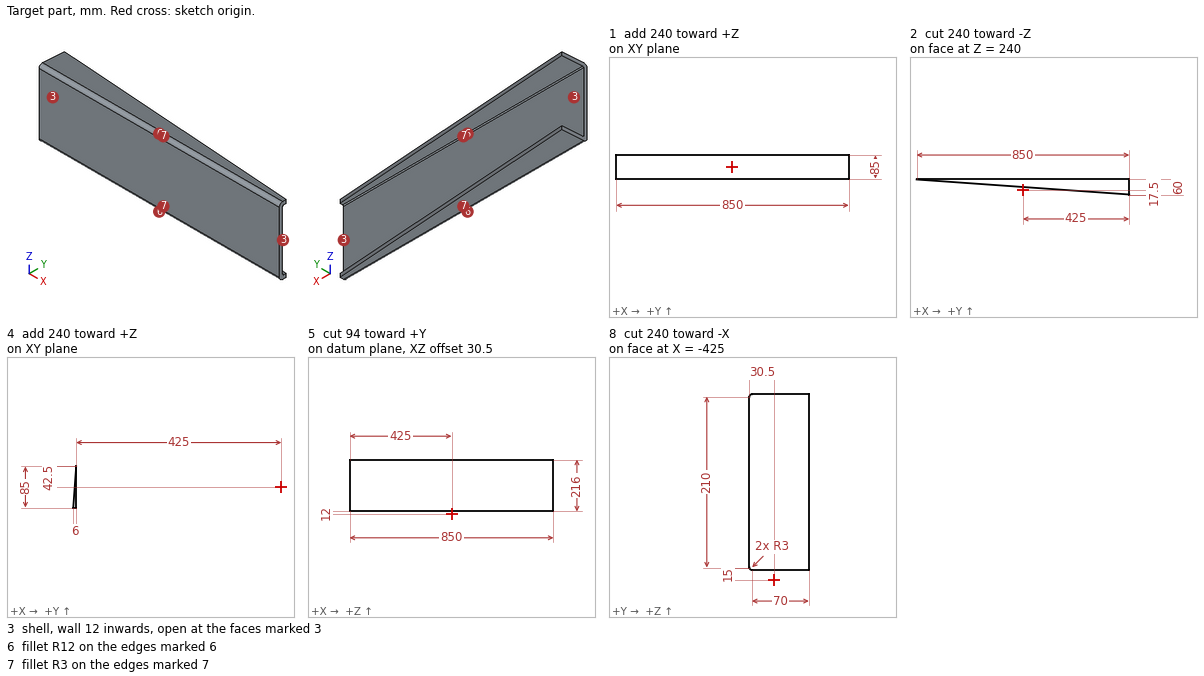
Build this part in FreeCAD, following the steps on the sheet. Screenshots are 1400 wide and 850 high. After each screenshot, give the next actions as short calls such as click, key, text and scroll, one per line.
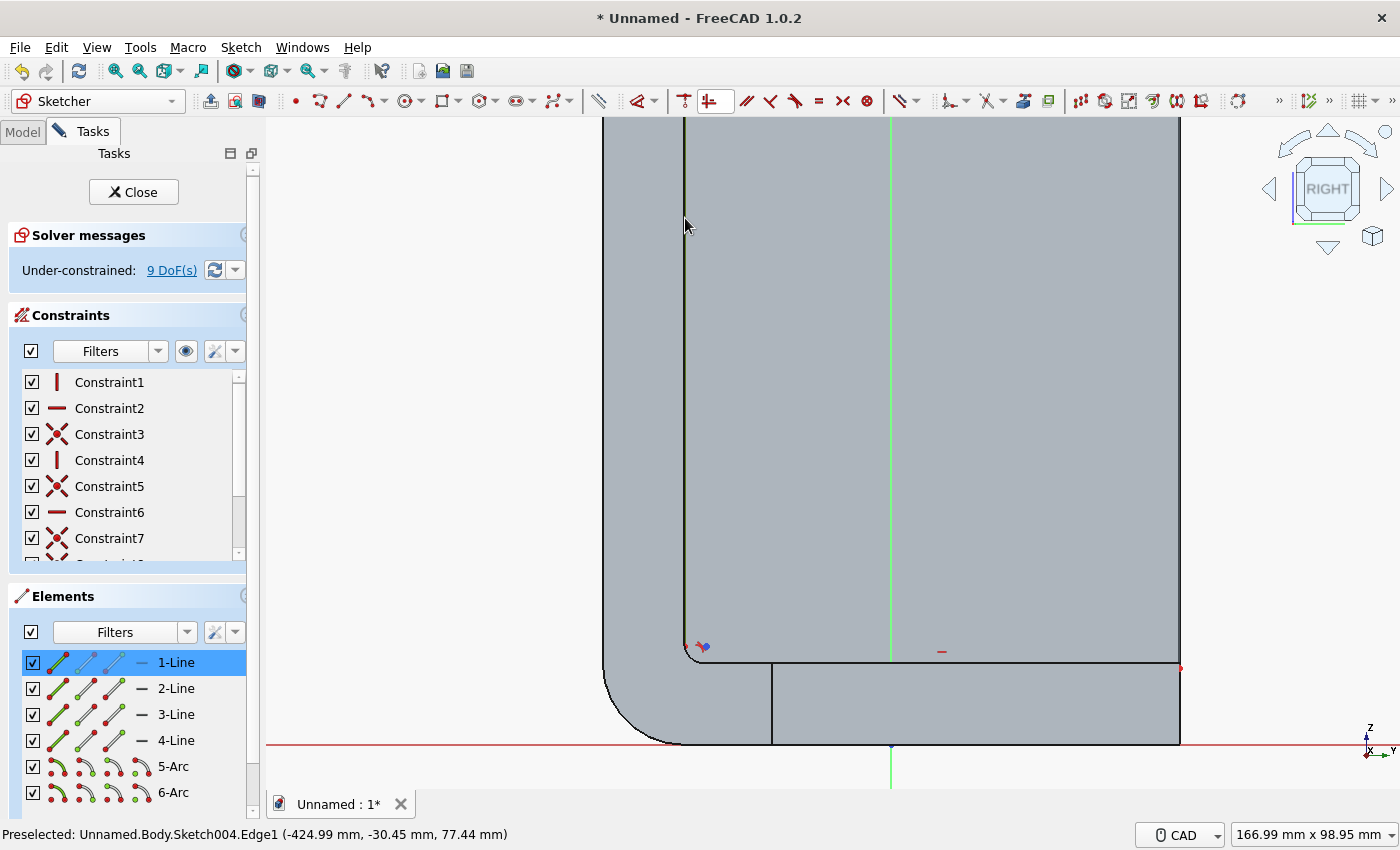
scroll(692, 661, down, 6)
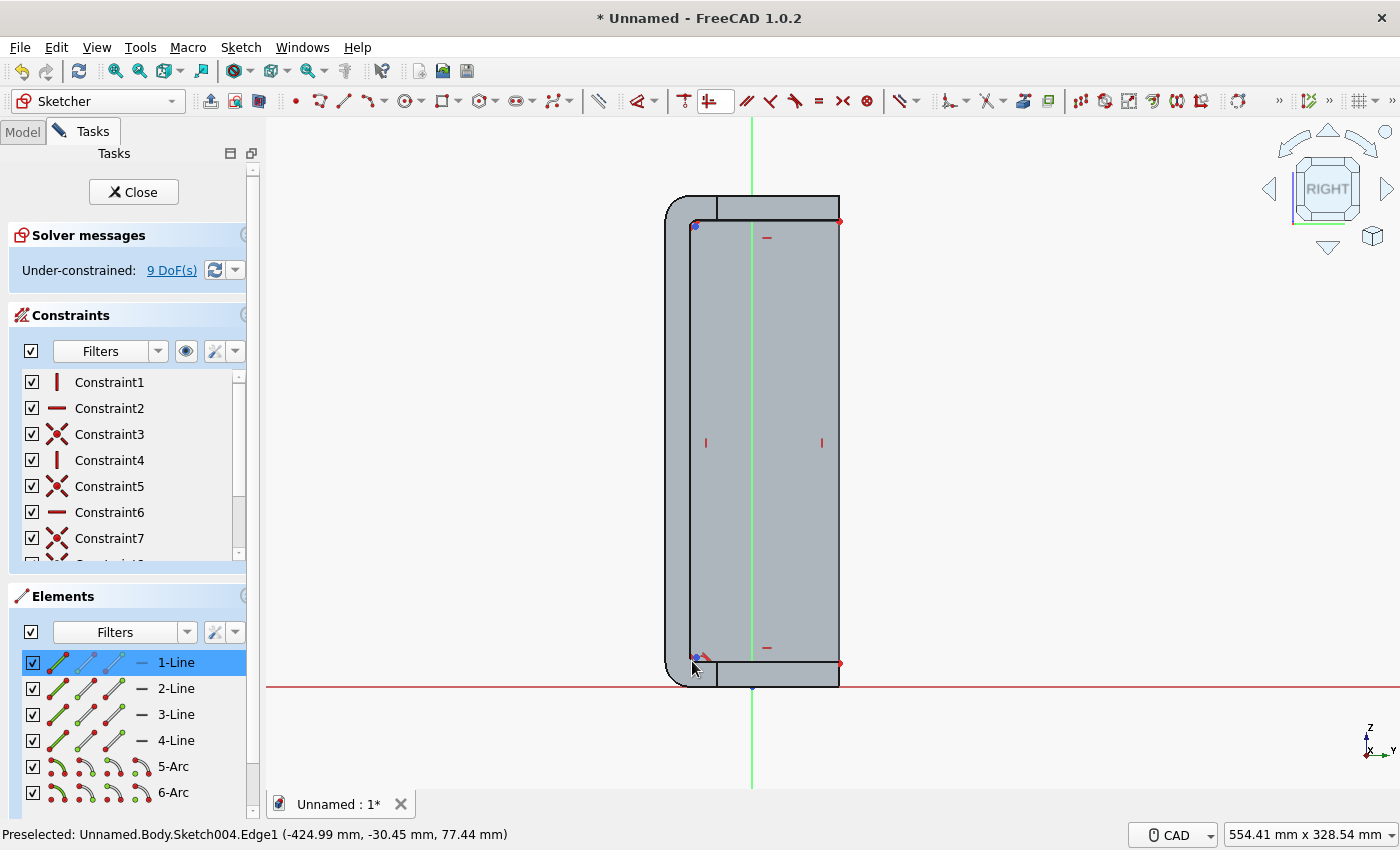
scroll(693, 222, up, 8)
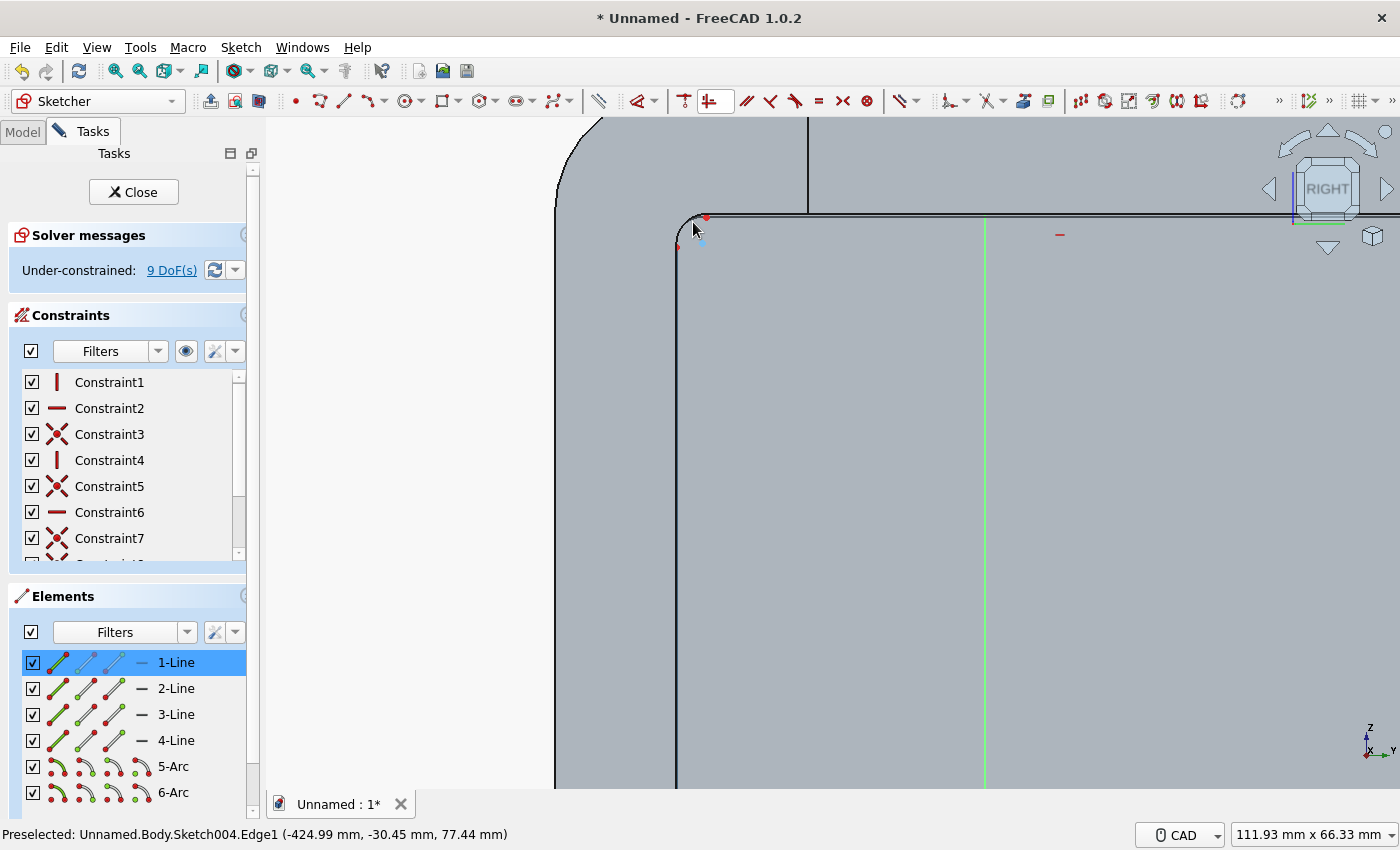
click(692, 219)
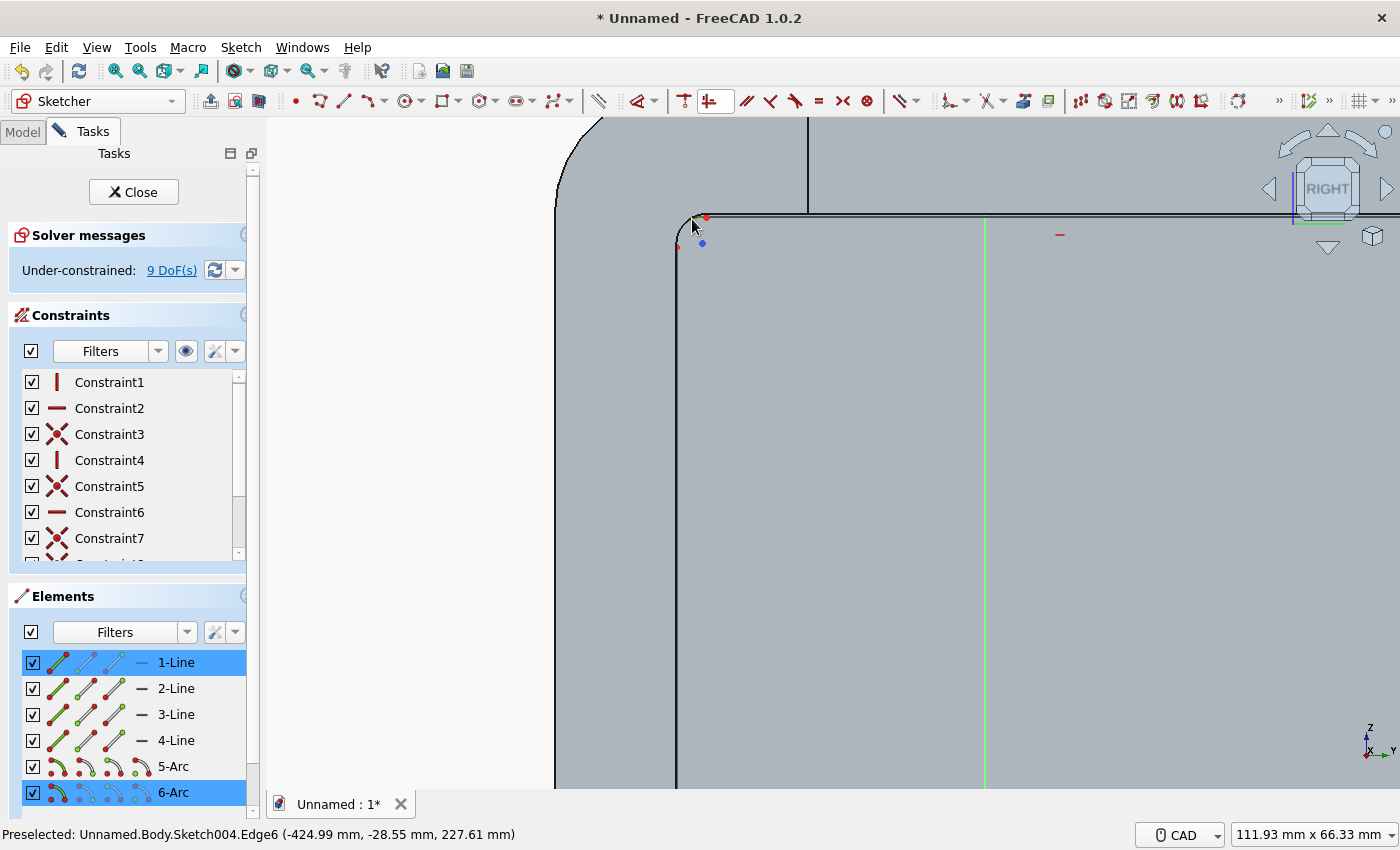
key(t)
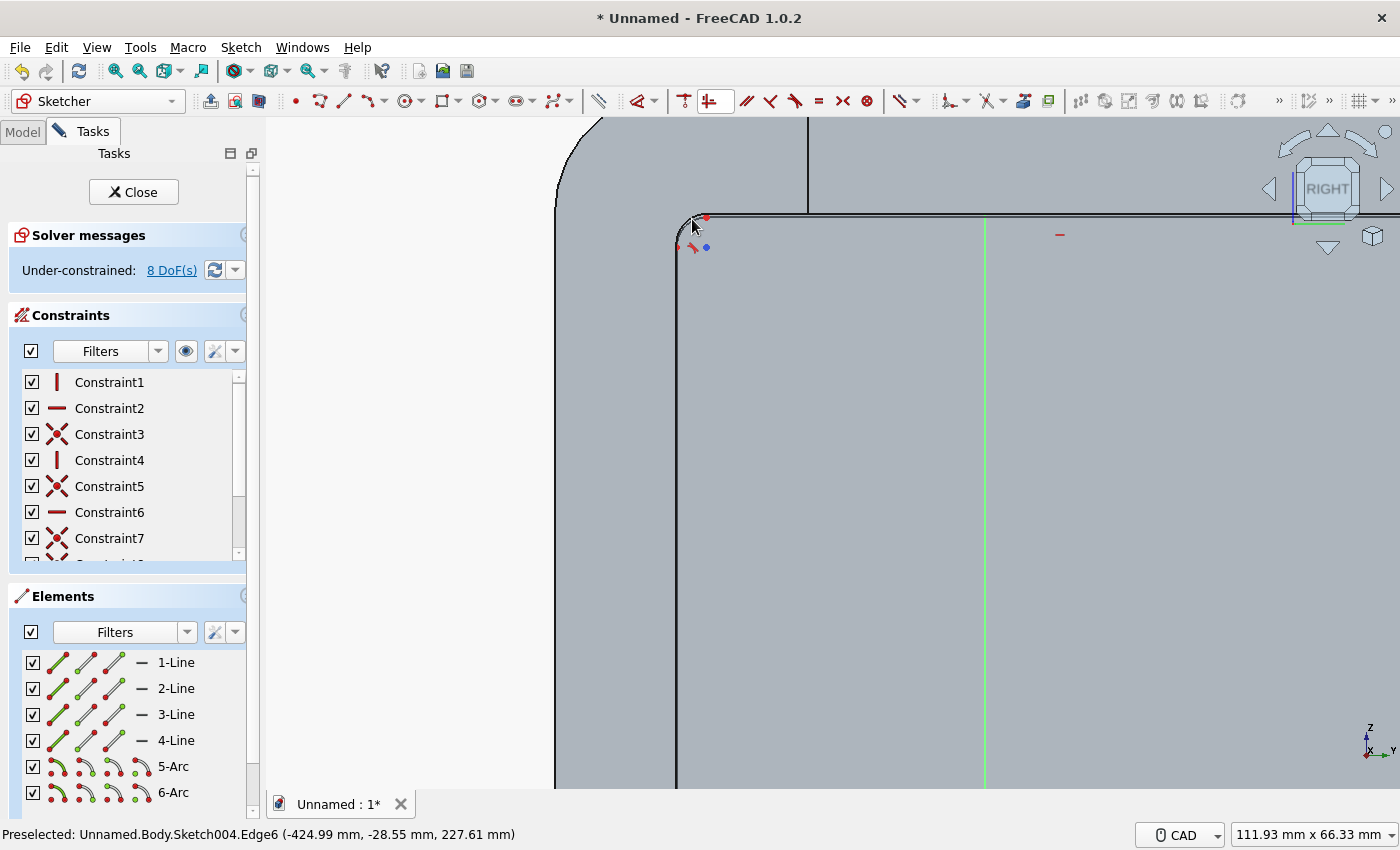
scroll(693, 221, down, 8)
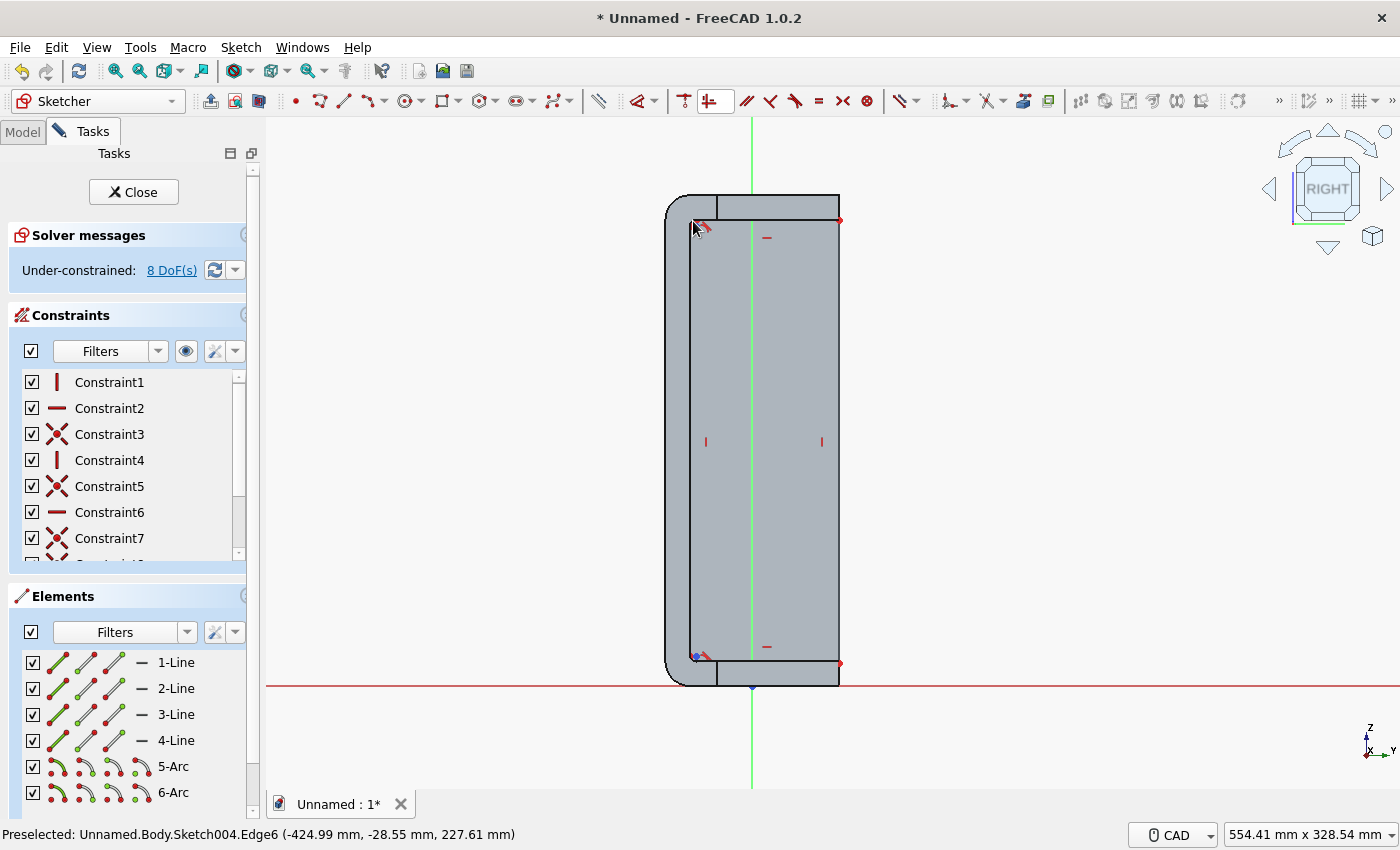
click(739, 663)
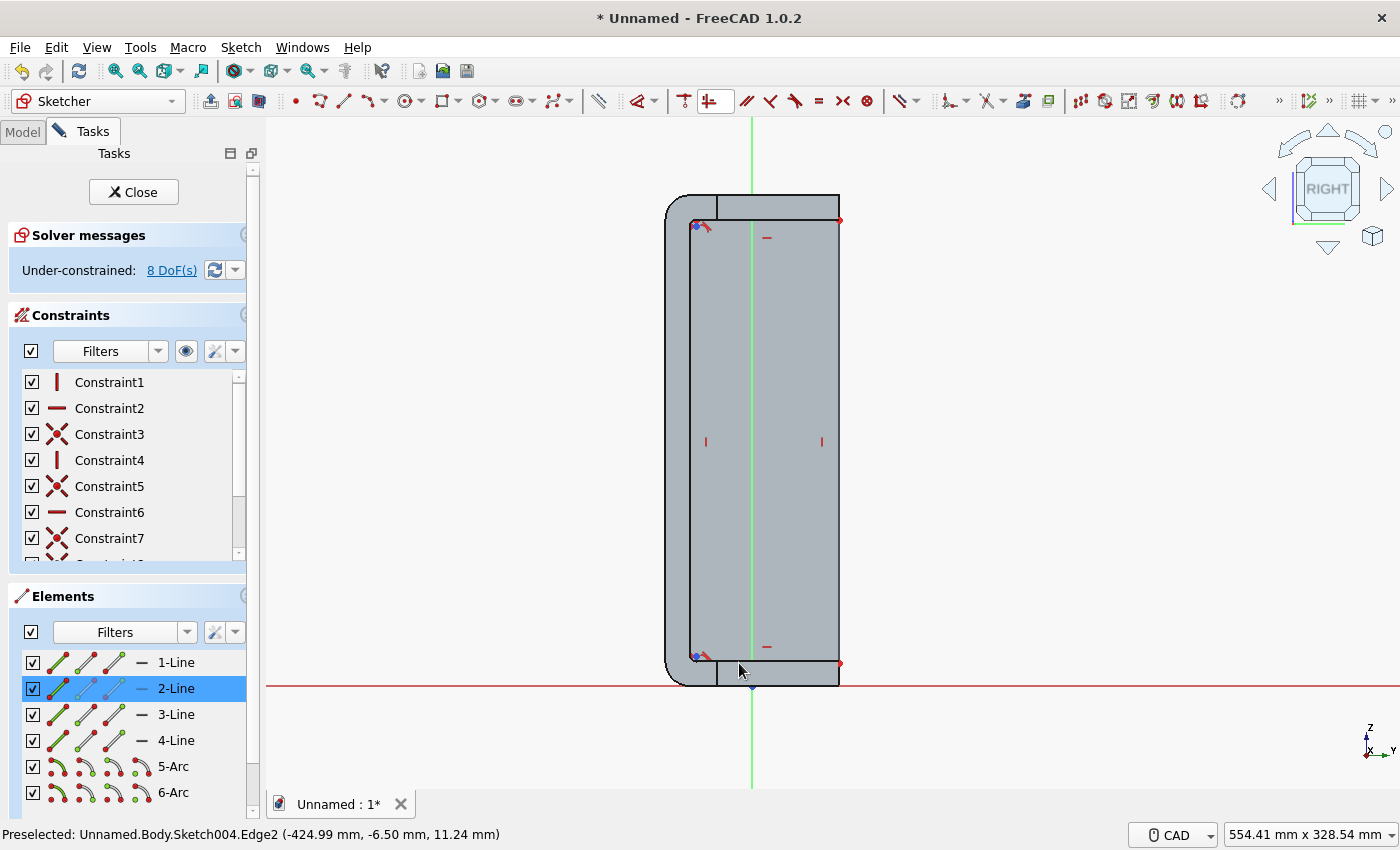
scroll(692, 661, up, 6)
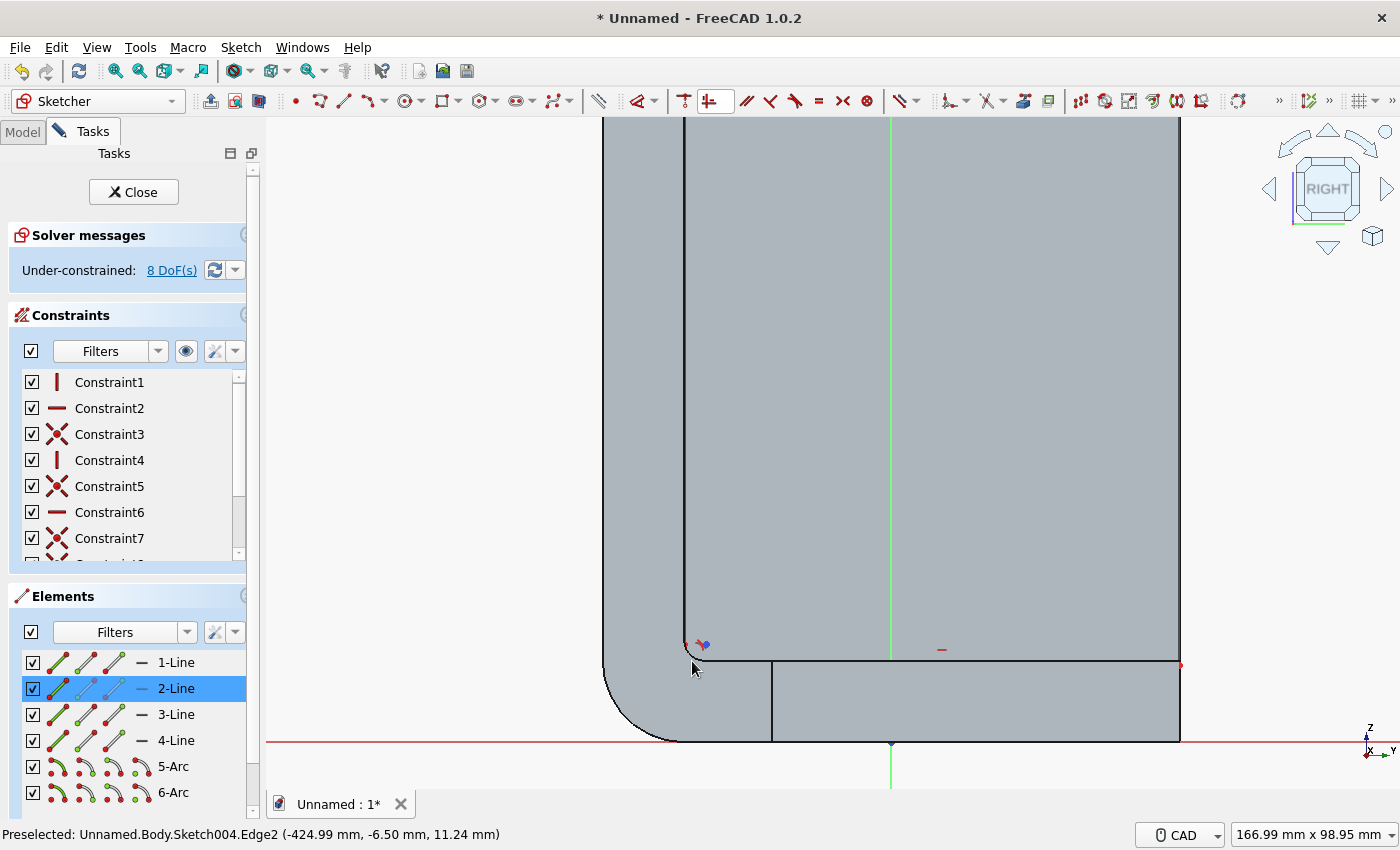
click(690, 659)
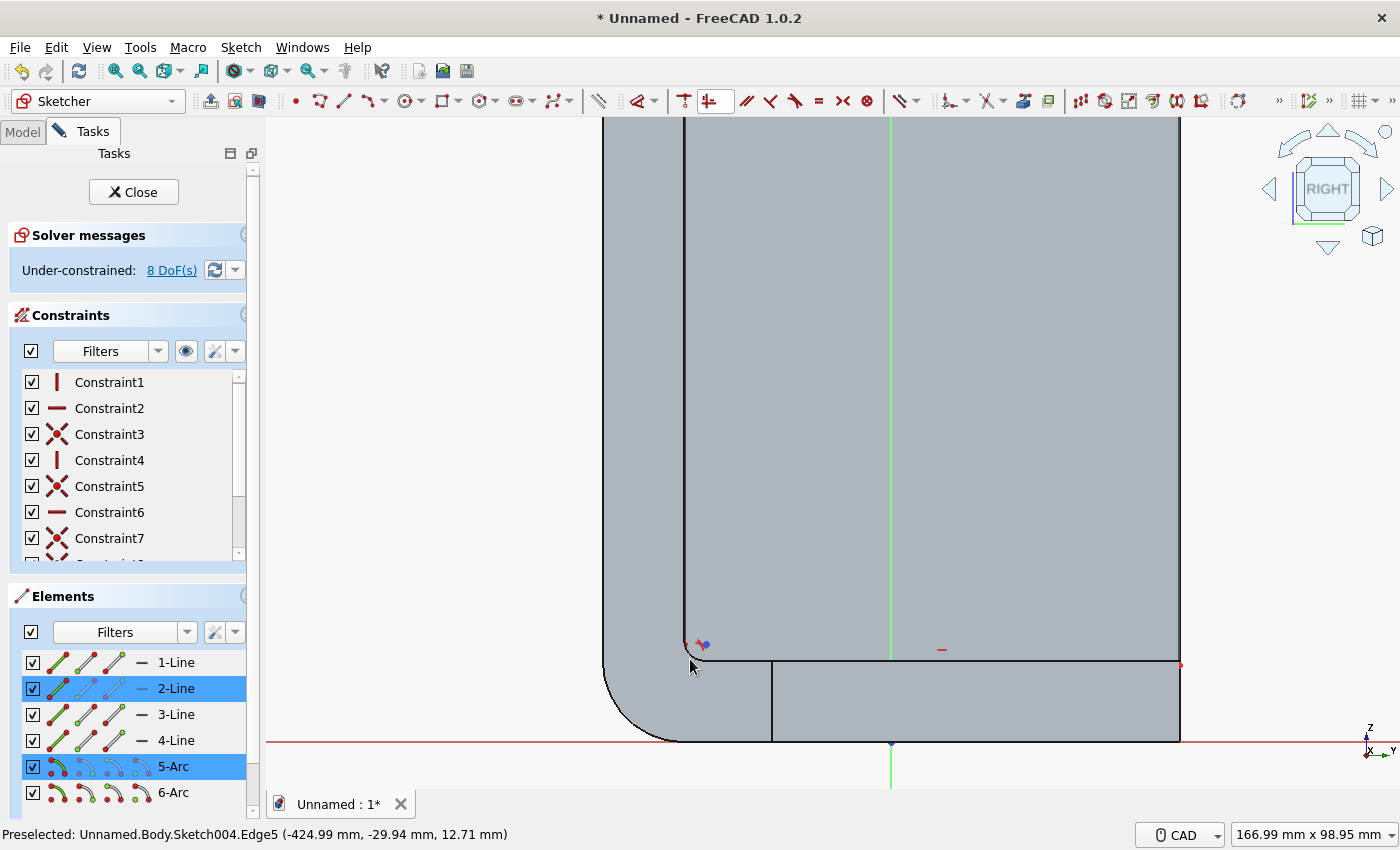
key(t)